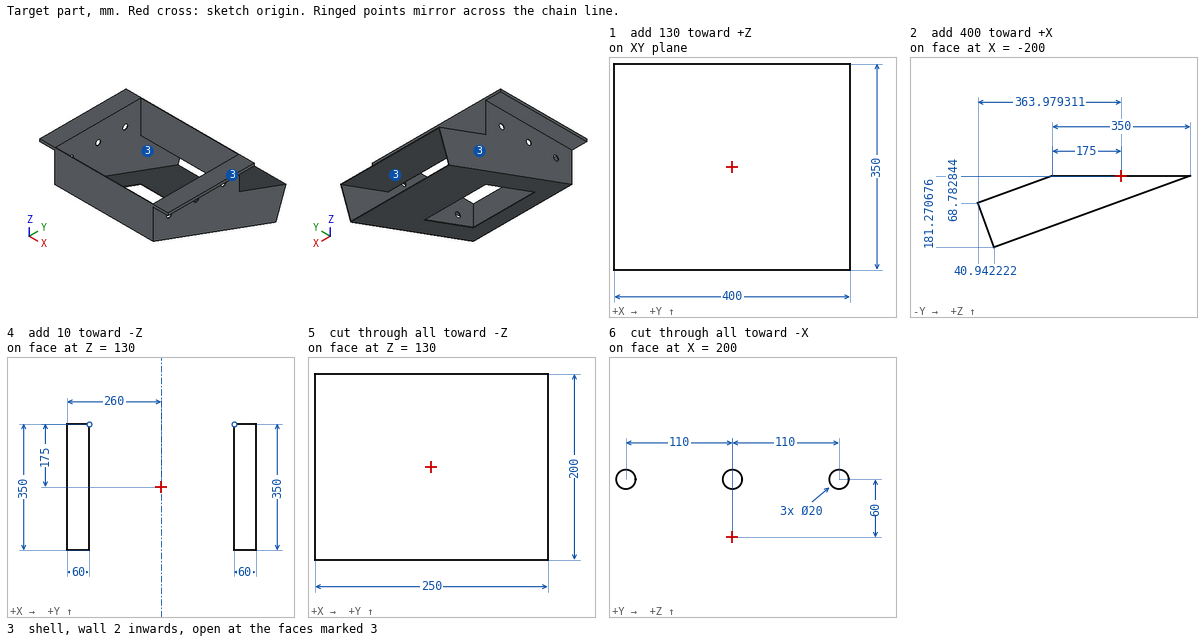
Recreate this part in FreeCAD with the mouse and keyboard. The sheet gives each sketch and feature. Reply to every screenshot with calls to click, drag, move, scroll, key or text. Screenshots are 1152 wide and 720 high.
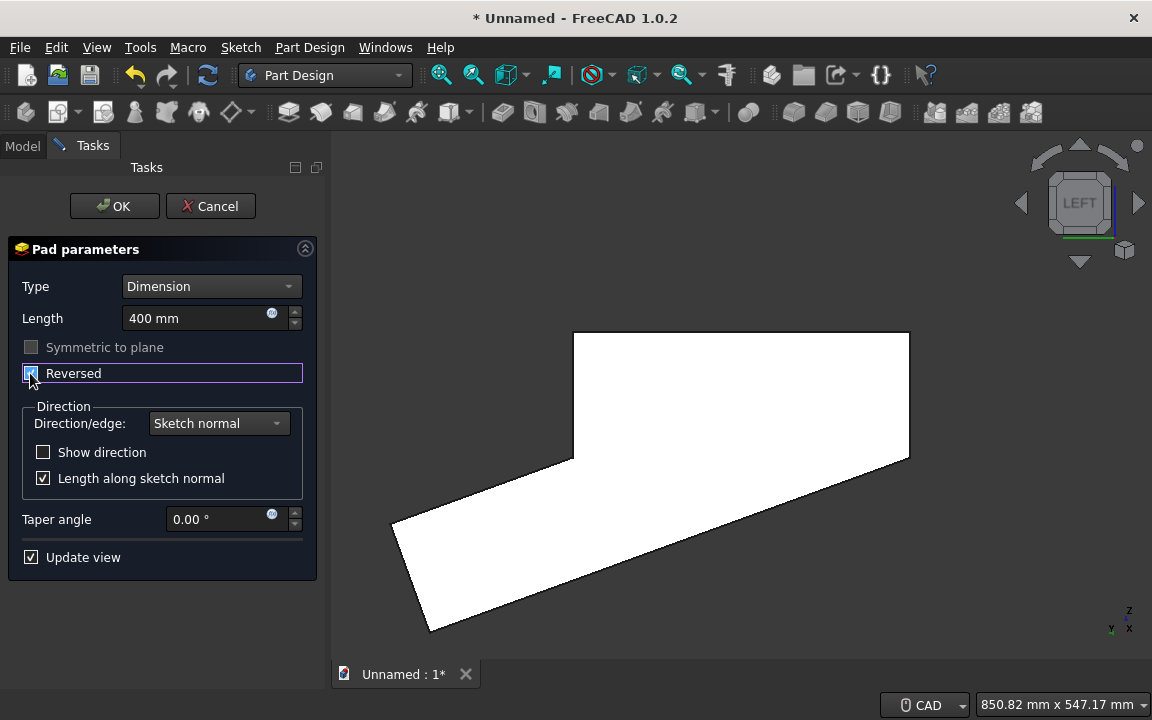
click(115, 206)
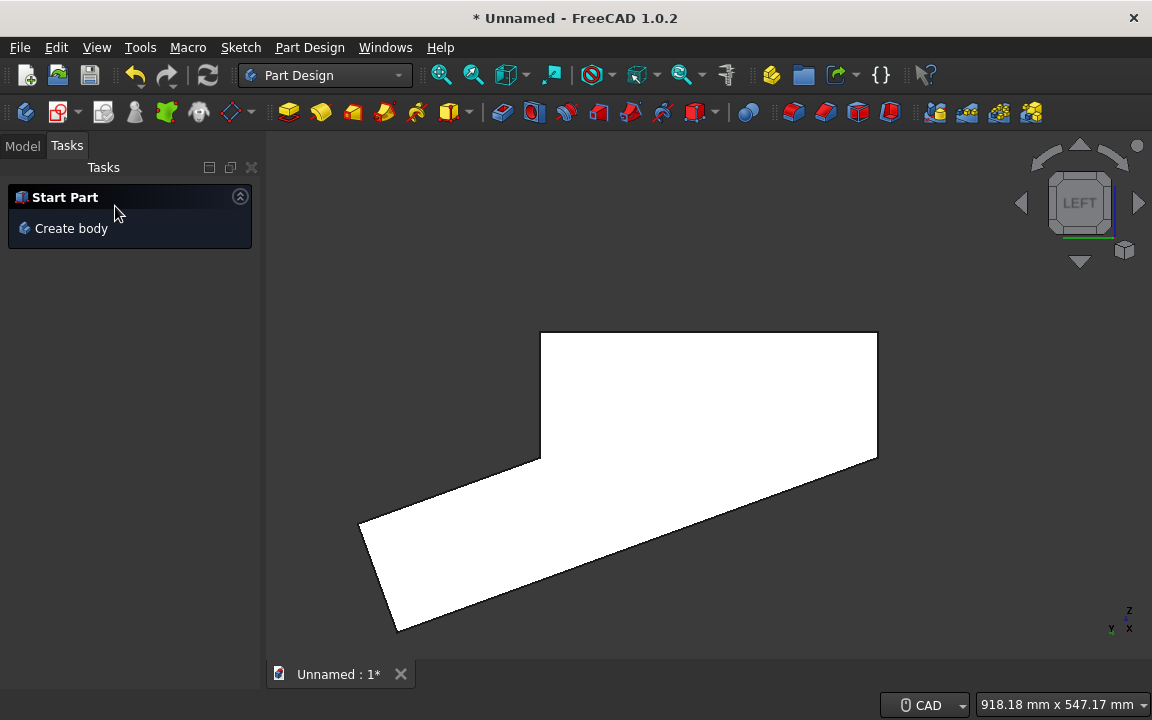
key(0)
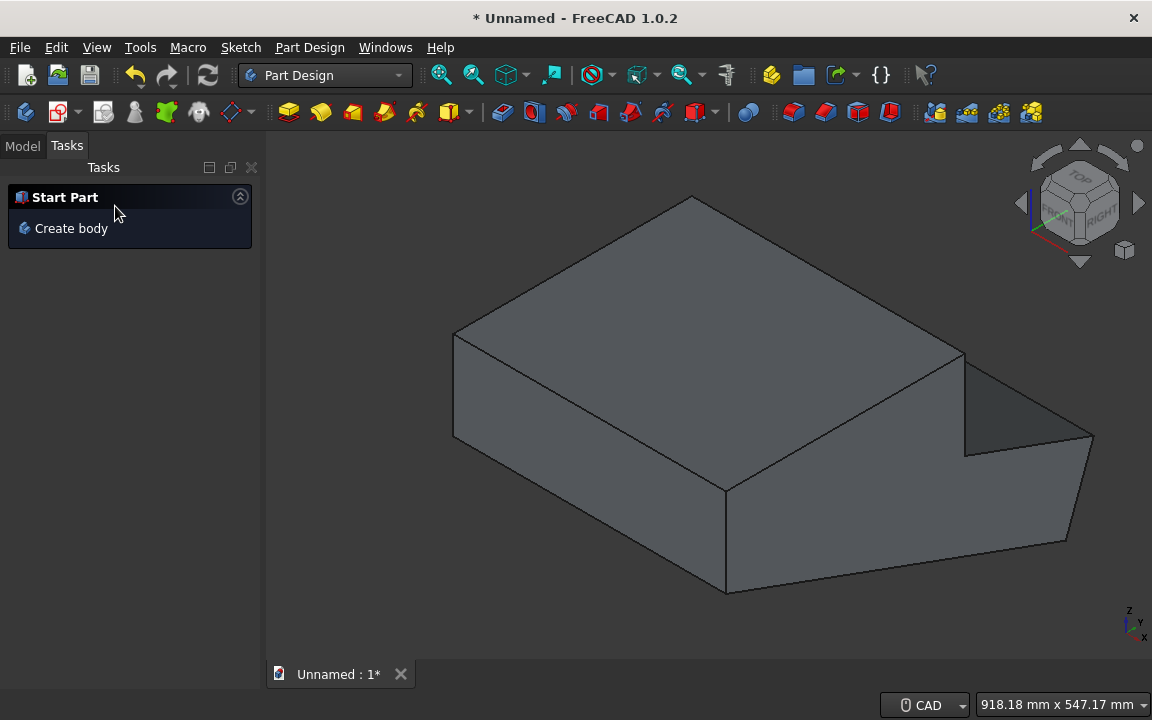
click(442, 76)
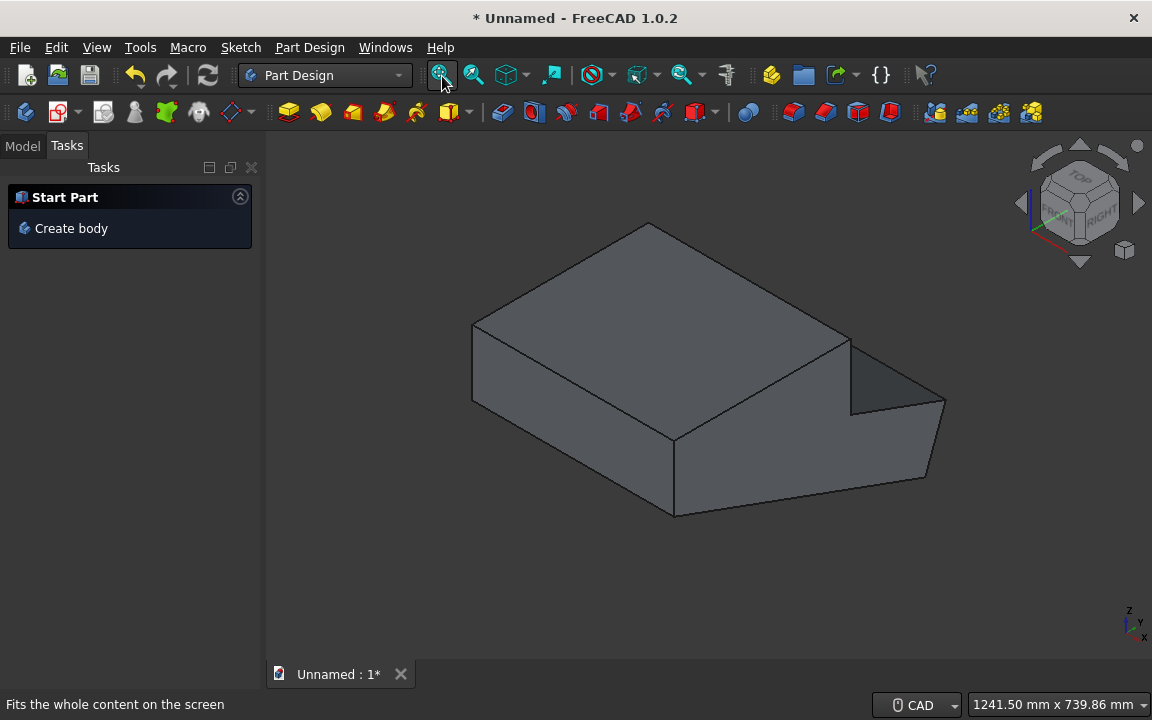
click(661, 331)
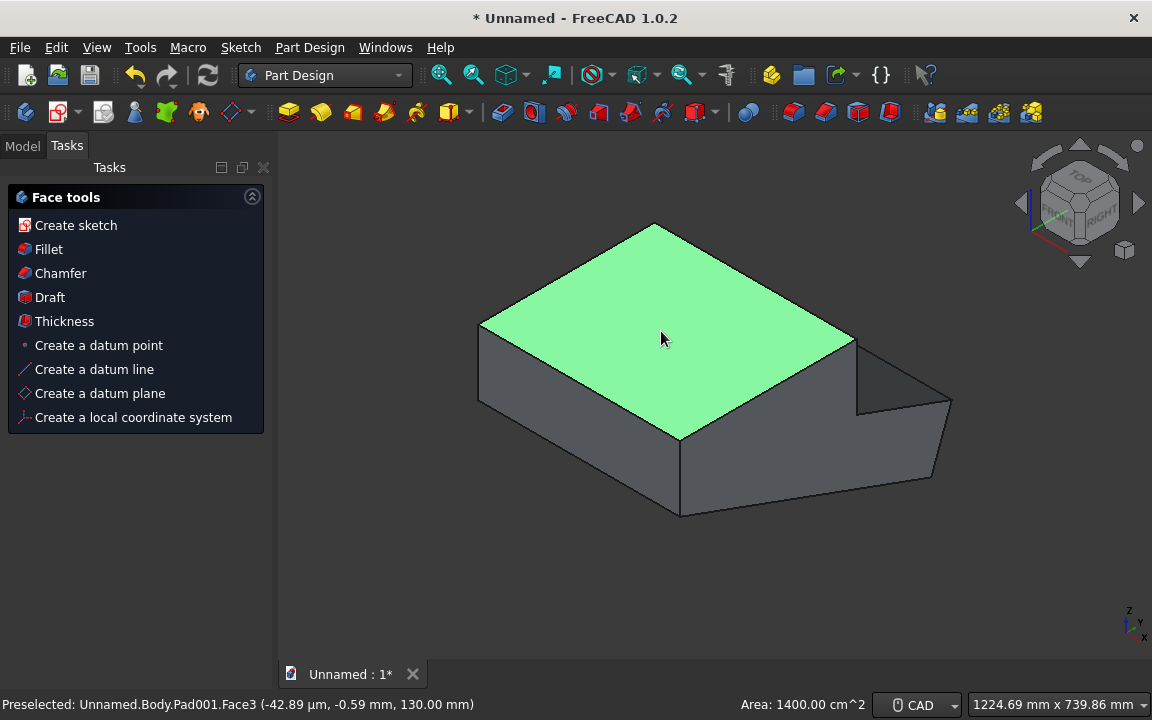
key(2)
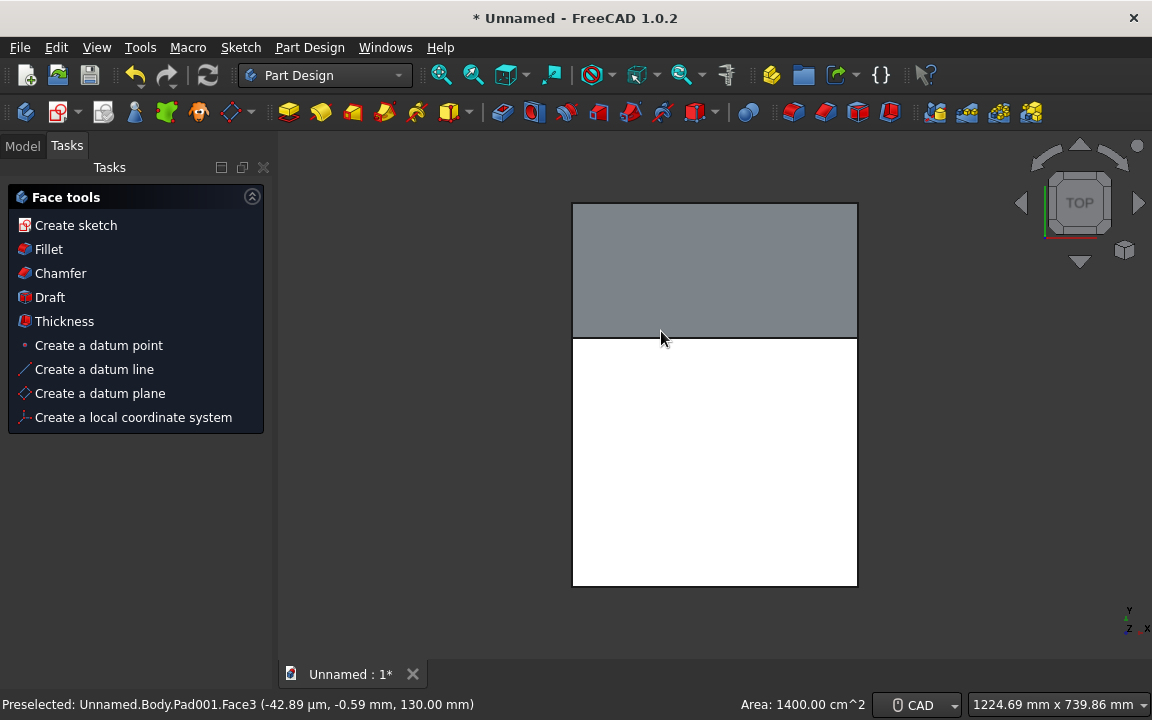
key(1)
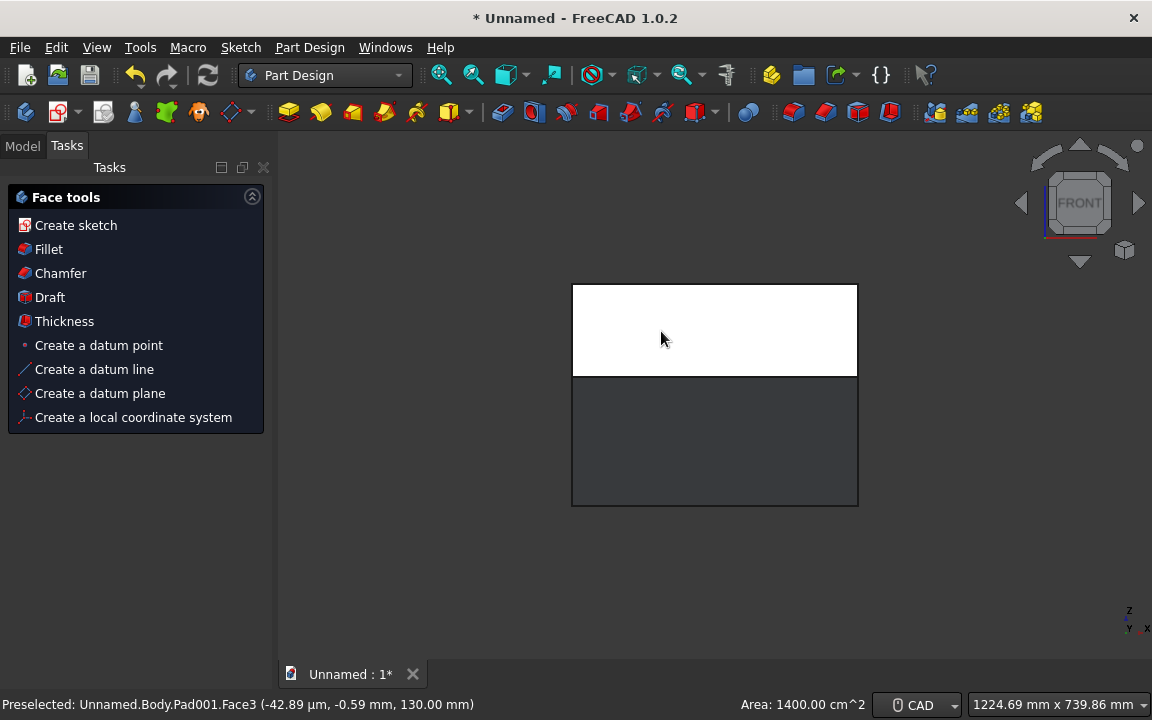
click(442, 76)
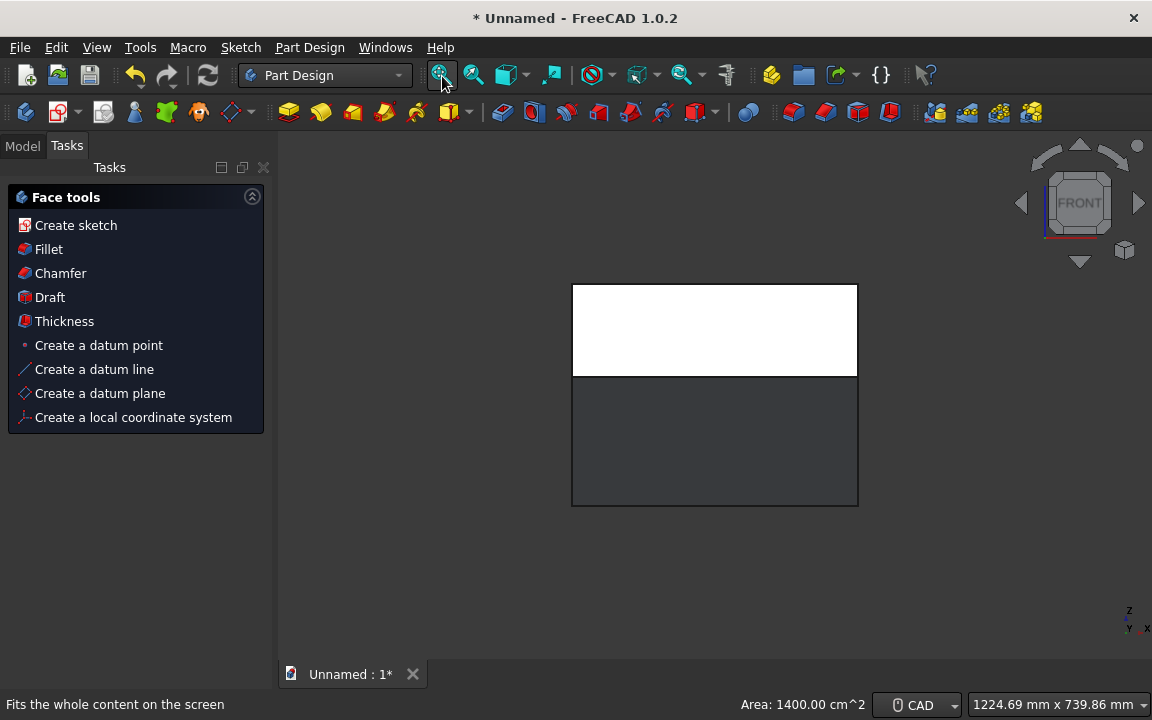
key(3)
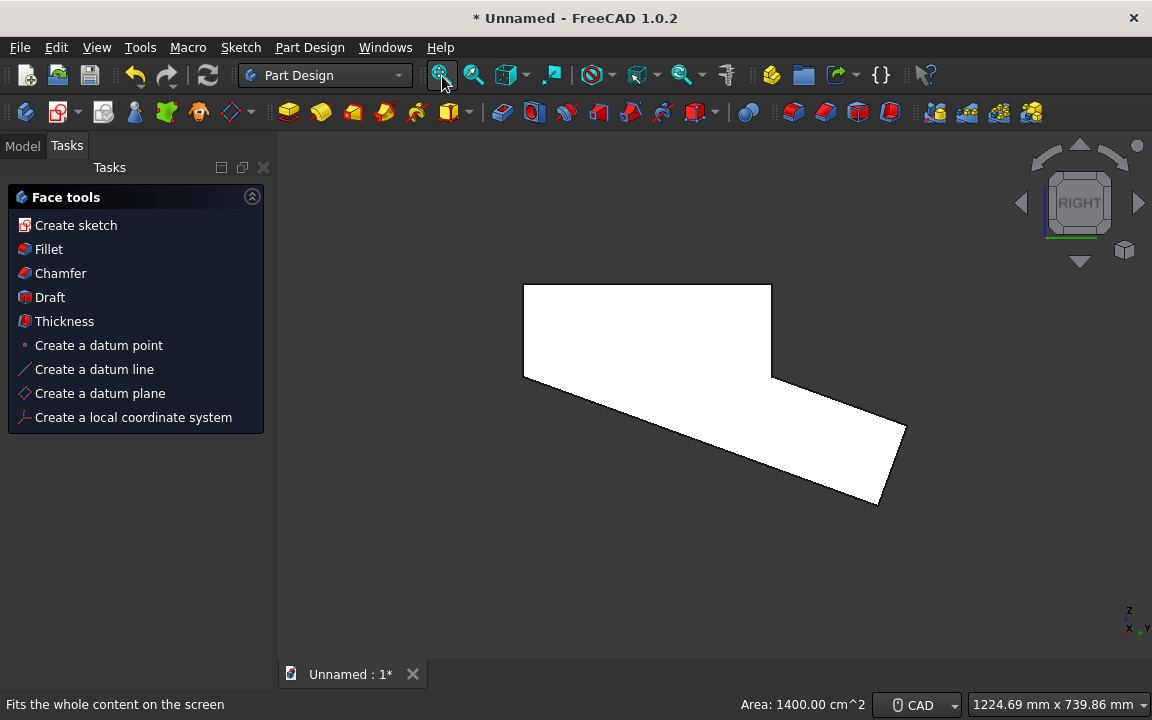
click(442, 76)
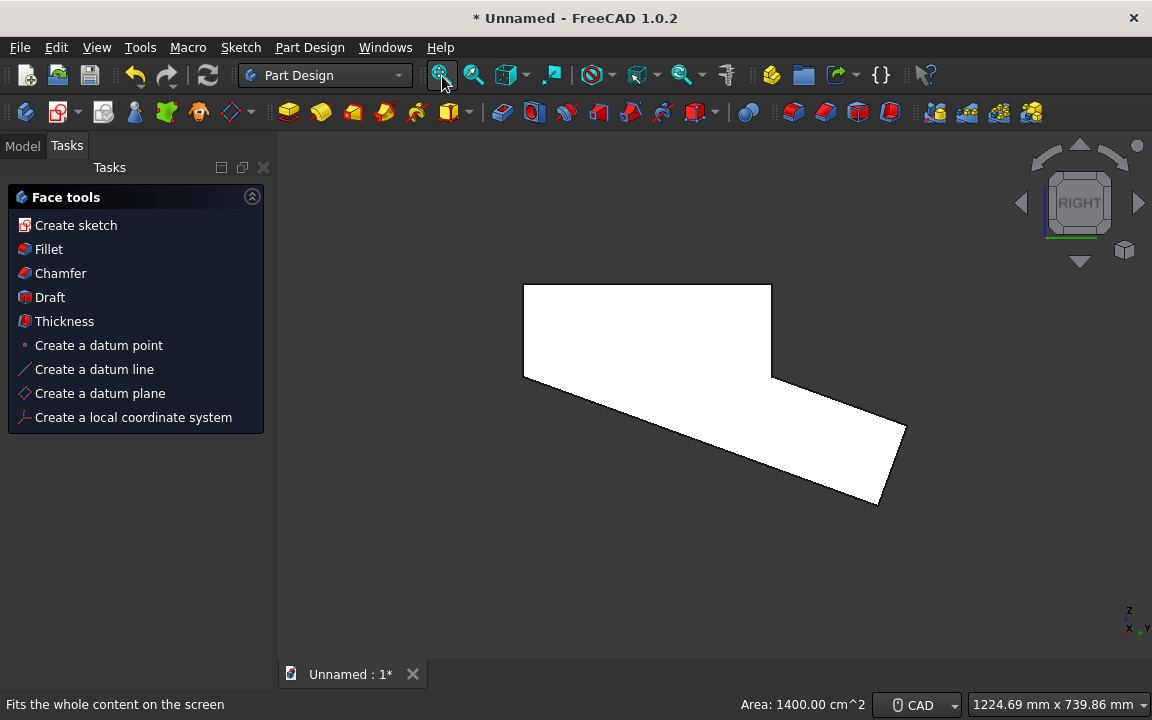
key(5)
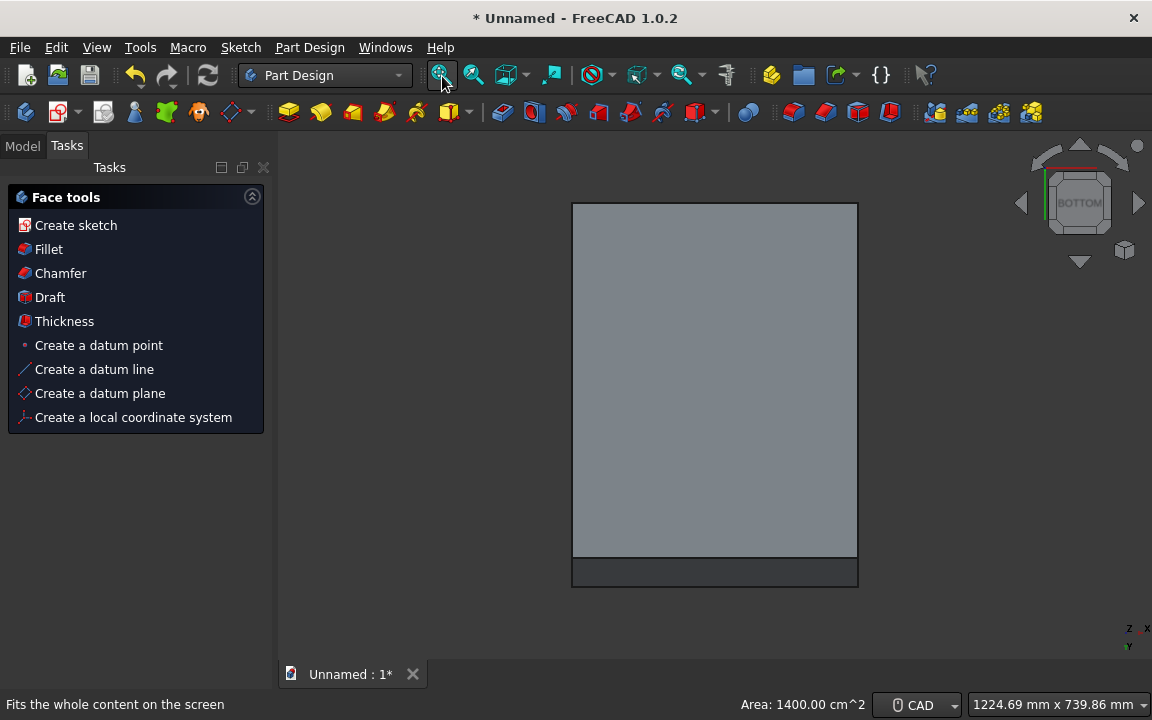
click(797, 572, ctrl)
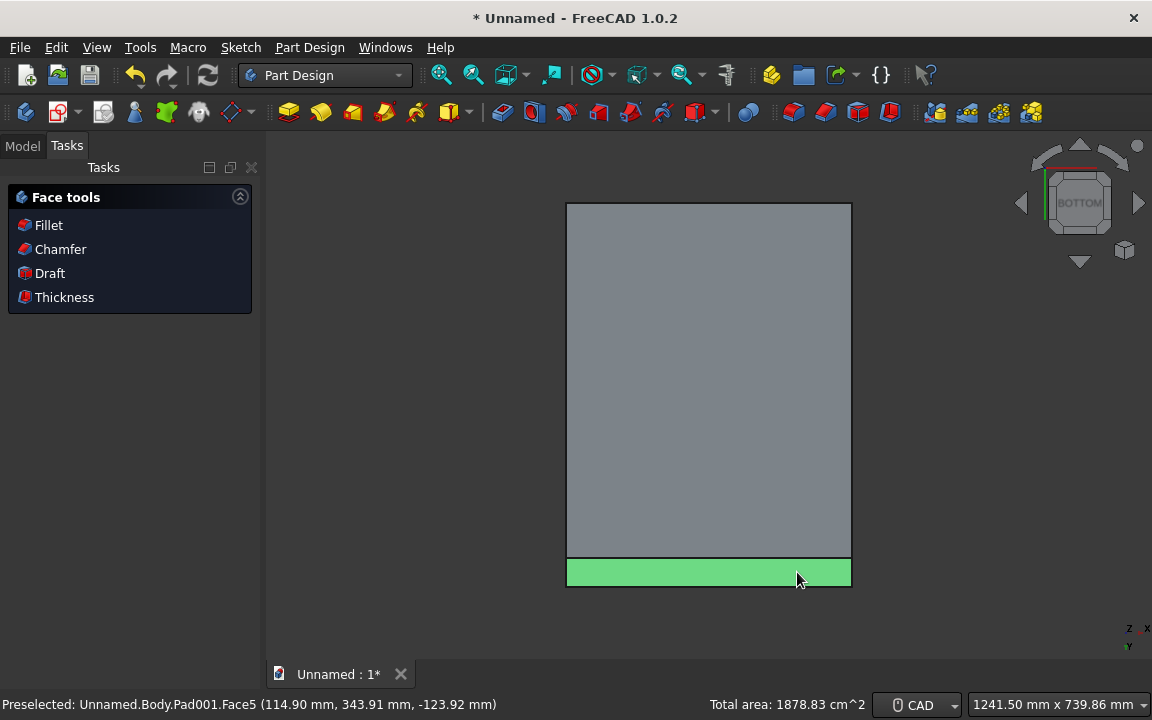
click(890, 112)